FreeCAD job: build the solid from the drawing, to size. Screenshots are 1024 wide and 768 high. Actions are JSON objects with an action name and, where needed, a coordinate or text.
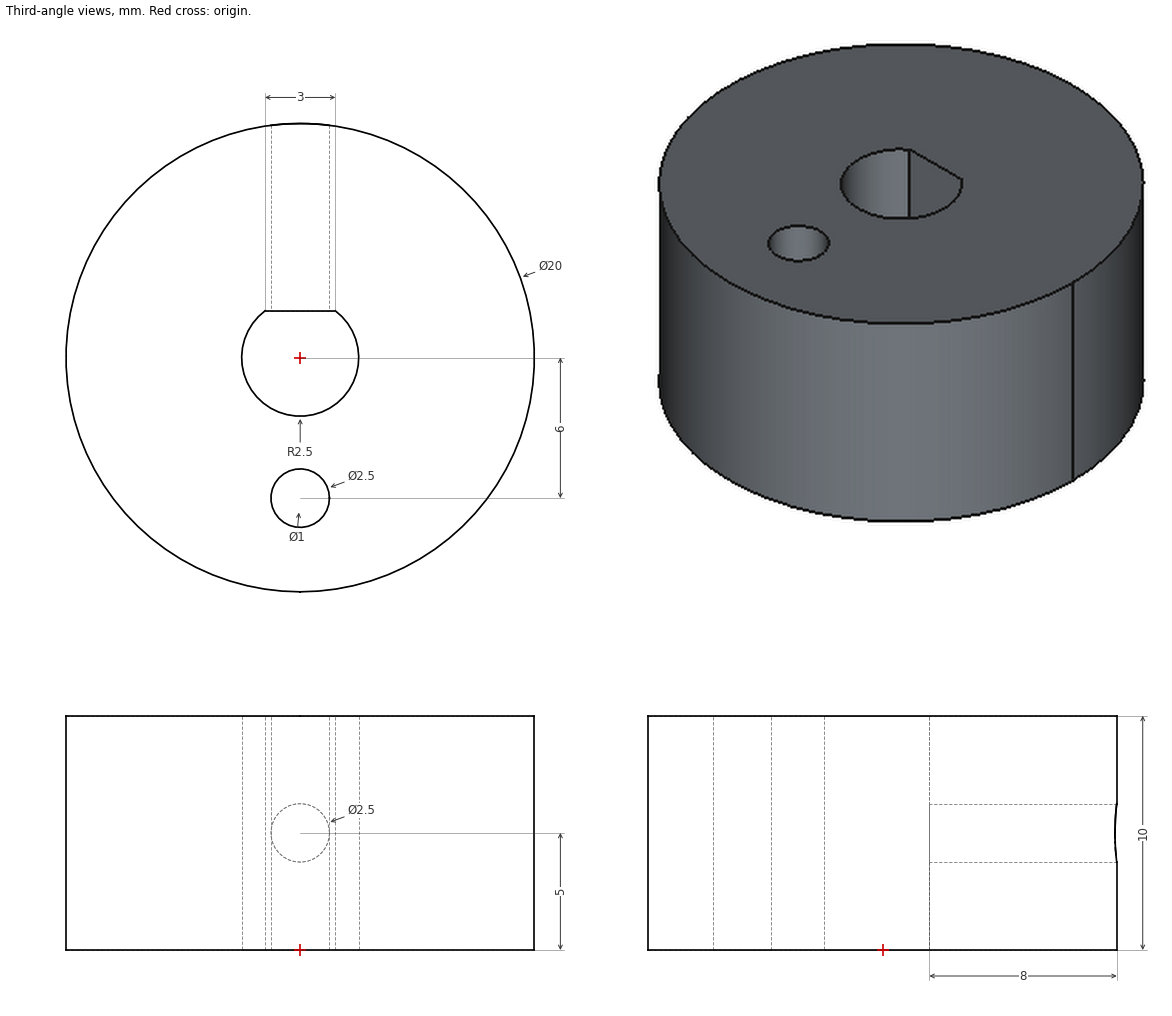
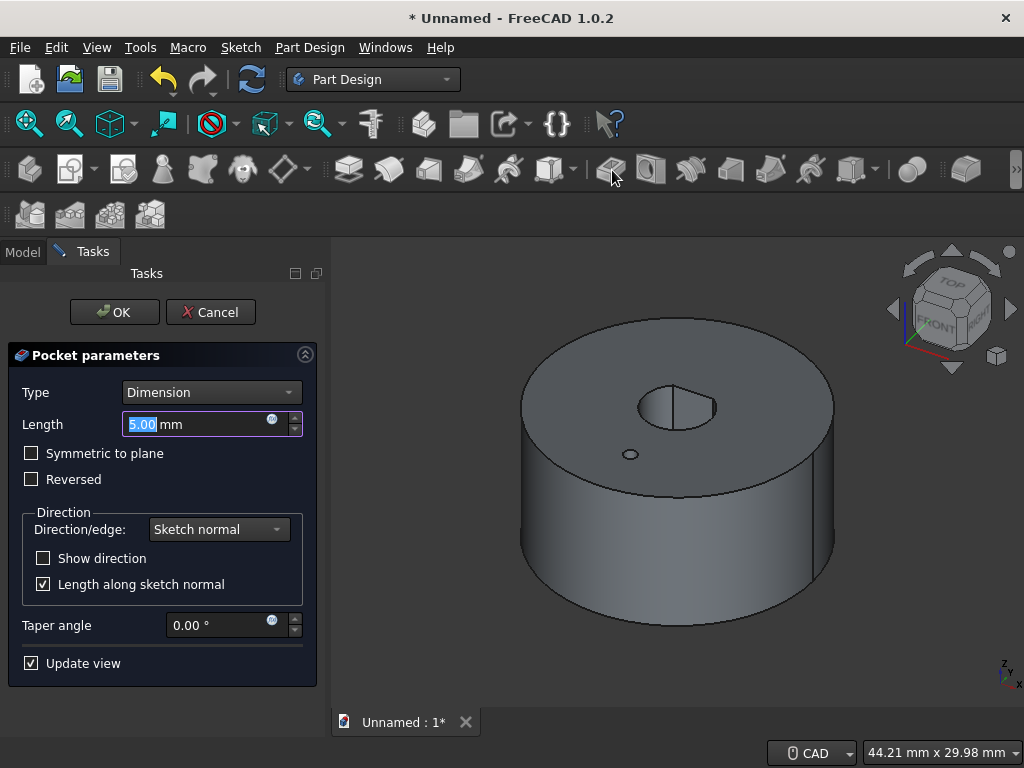
{"action": "left_click", "coordinate": [212, 392]}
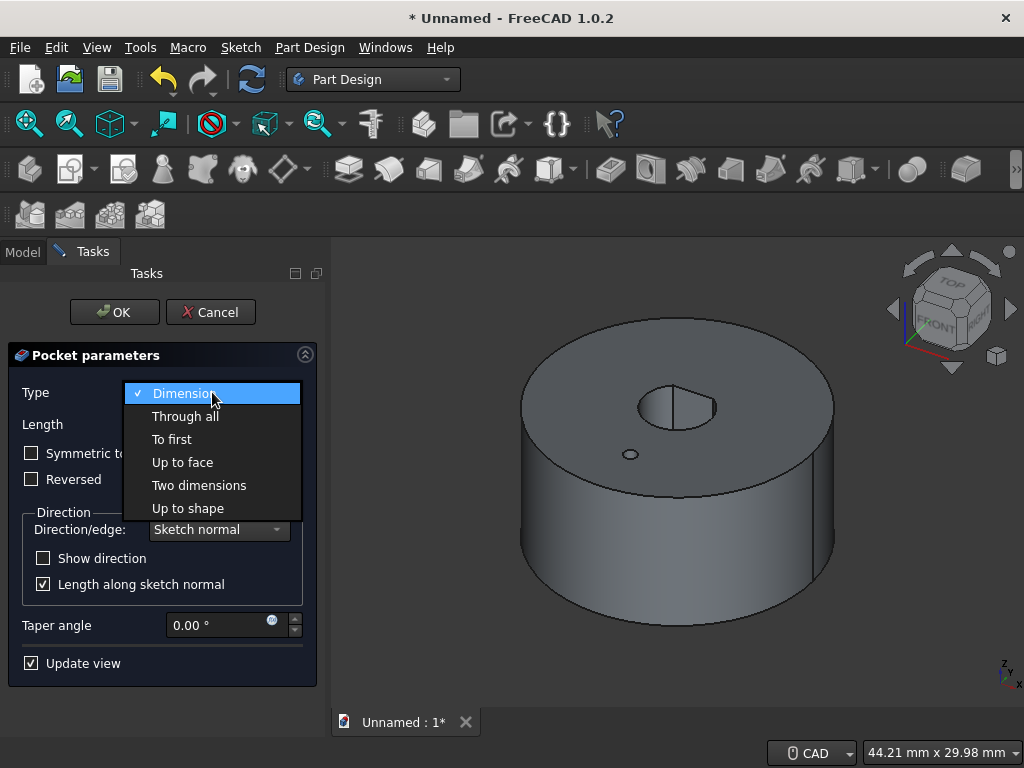
{"action": "left_click", "coordinate": [212, 416]}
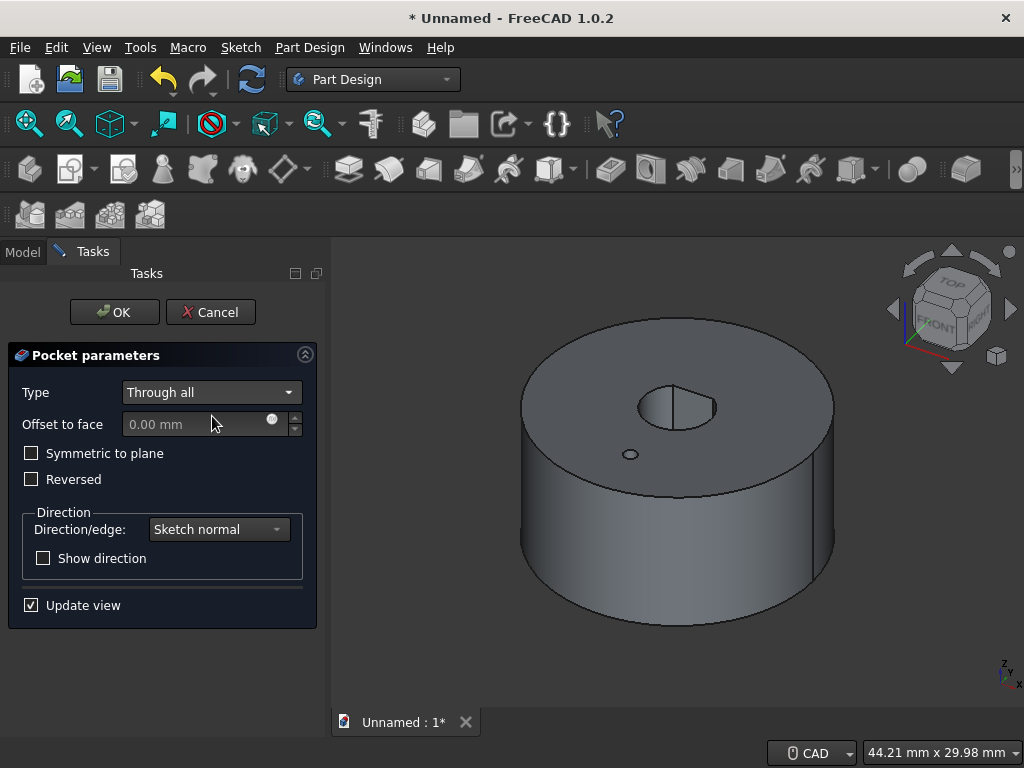
{"action": "left_click", "coordinate": [115, 312]}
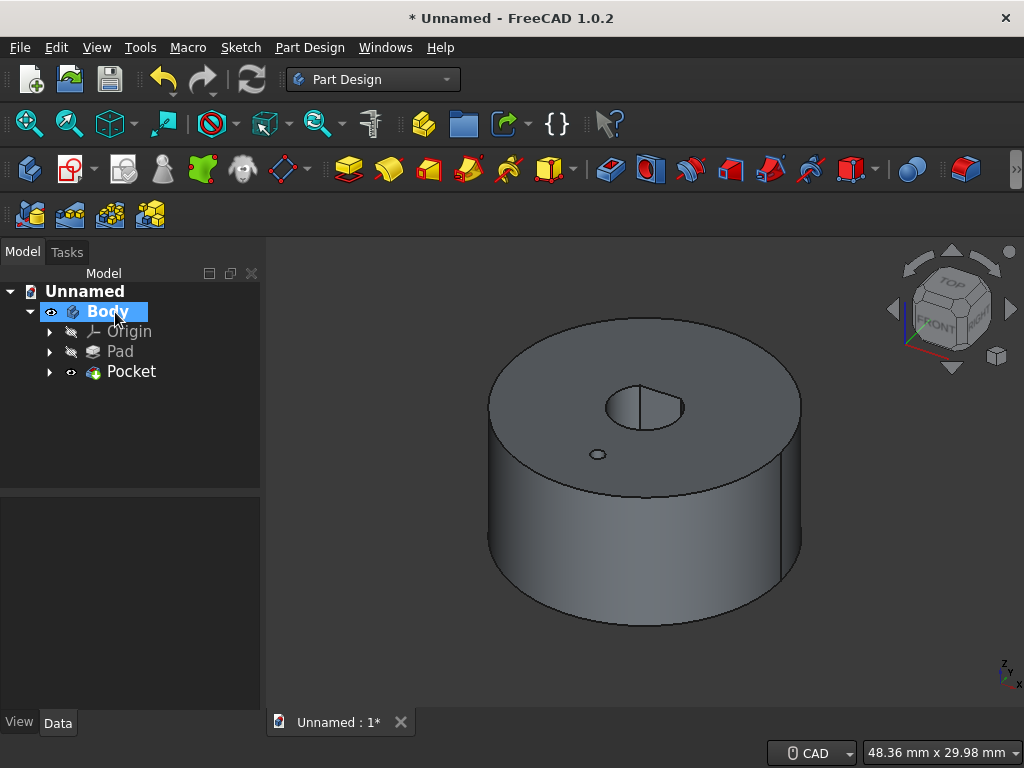
{"action": "left_click", "coordinate": [50, 332]}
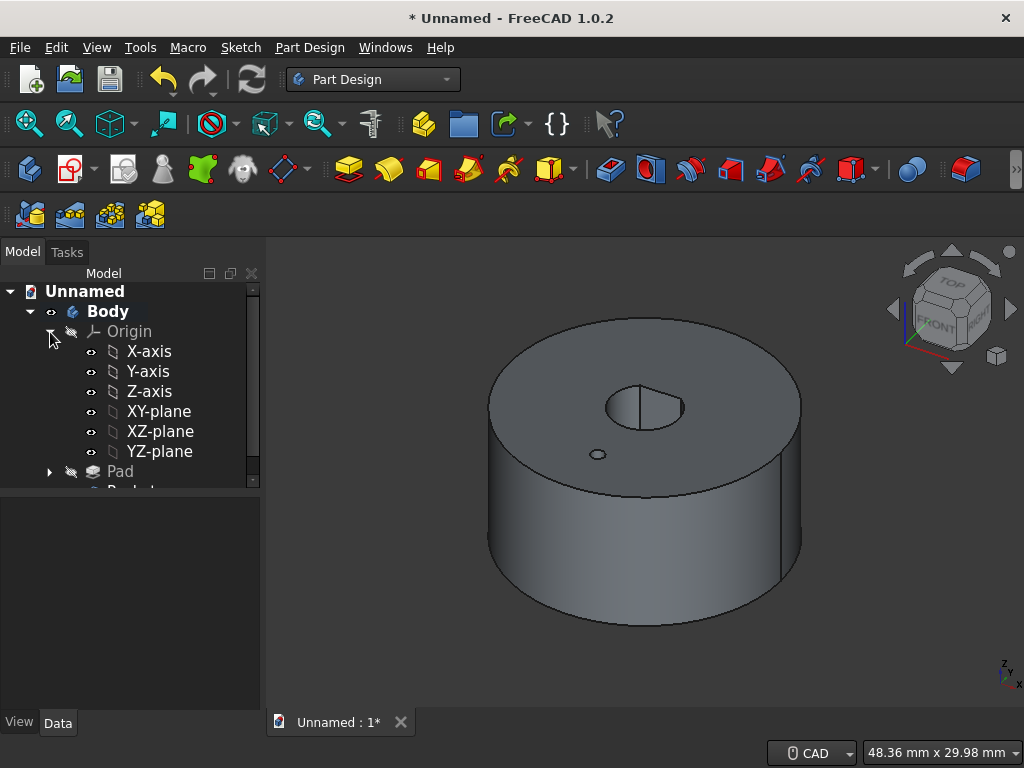
{"action": "left_click", "coordinate": [136, 432]}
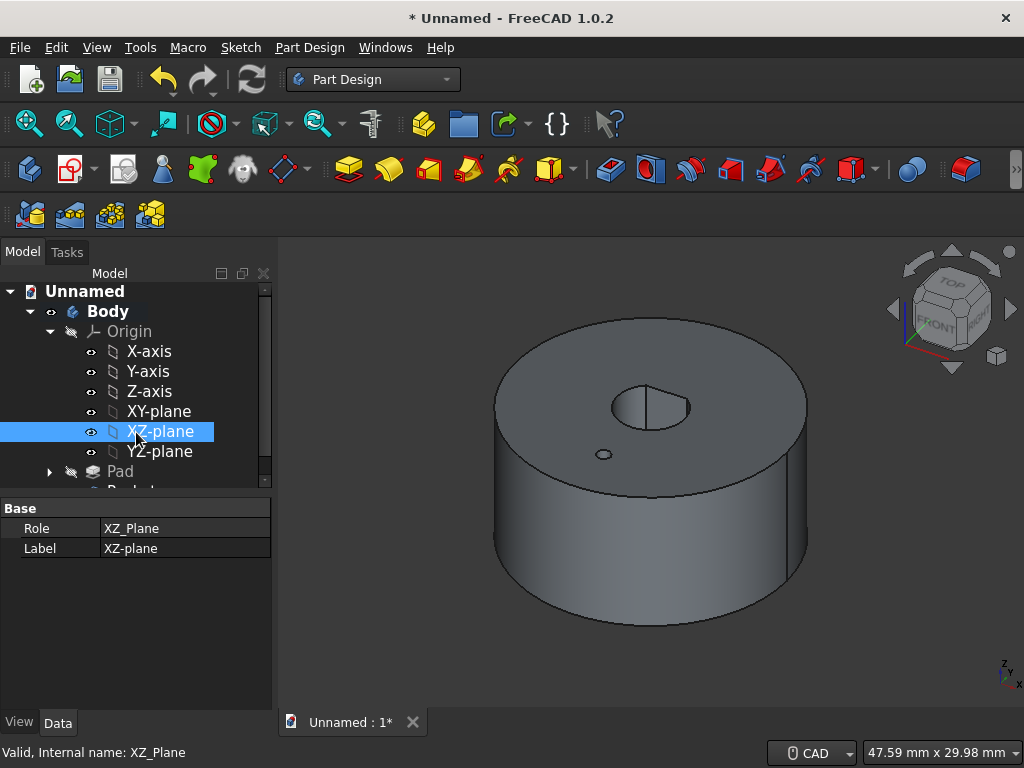
{"action": "left_click", "coordinate": [284, 170]}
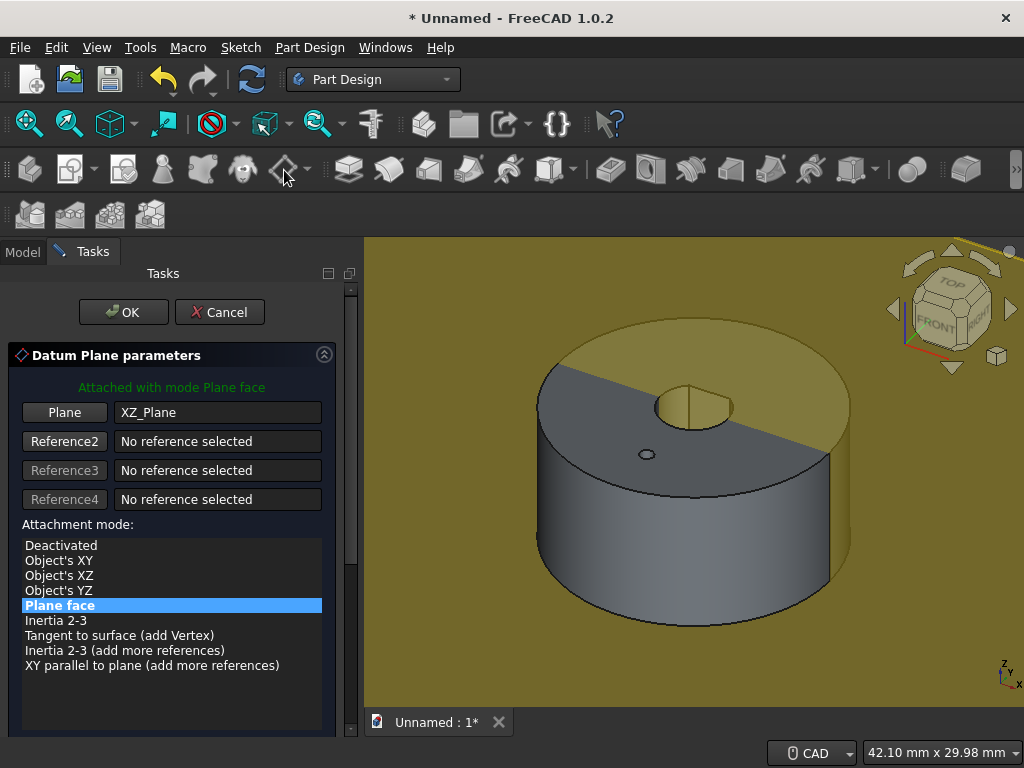
{"action": "scroll", "coordinate": [351, 510], "scroll_direction": "down", "scroll_amount": 3}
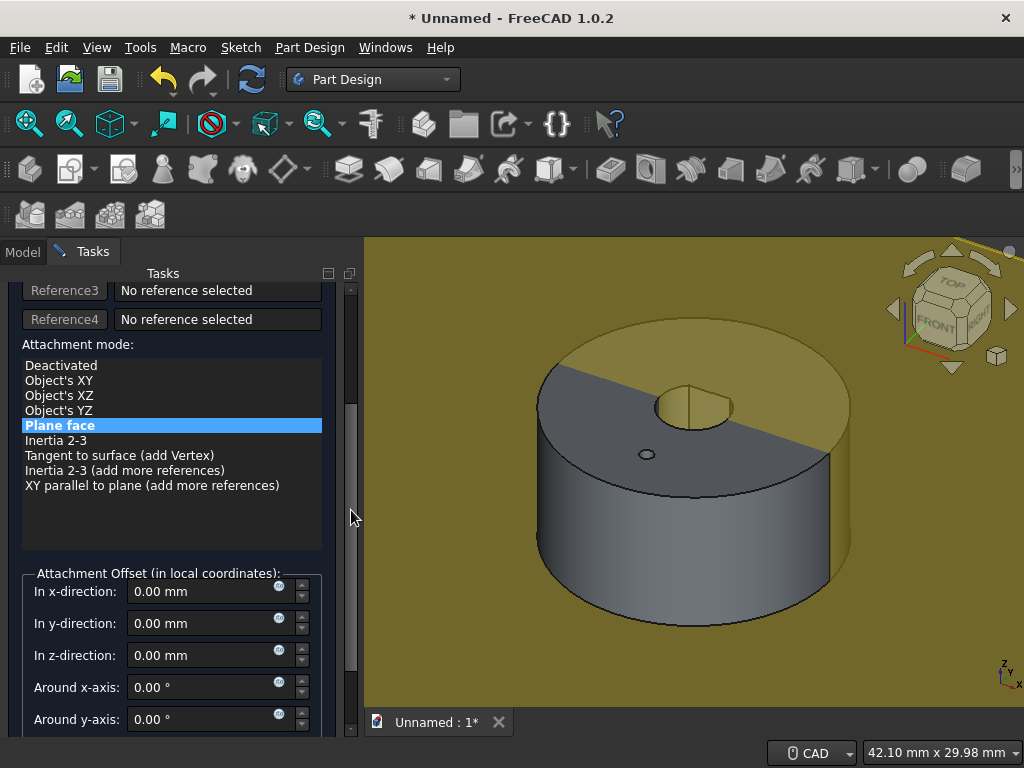
{"action": "triple_click", "coordinate": [210, 655]}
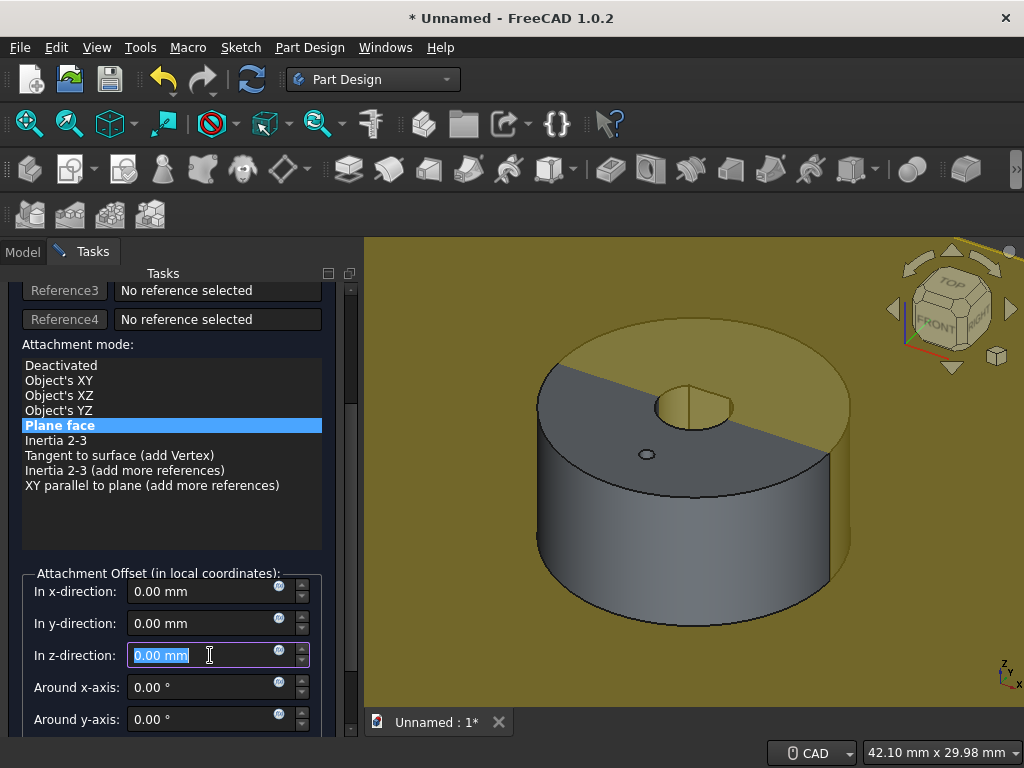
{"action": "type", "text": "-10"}
{"action": "key", "text": "Tab"}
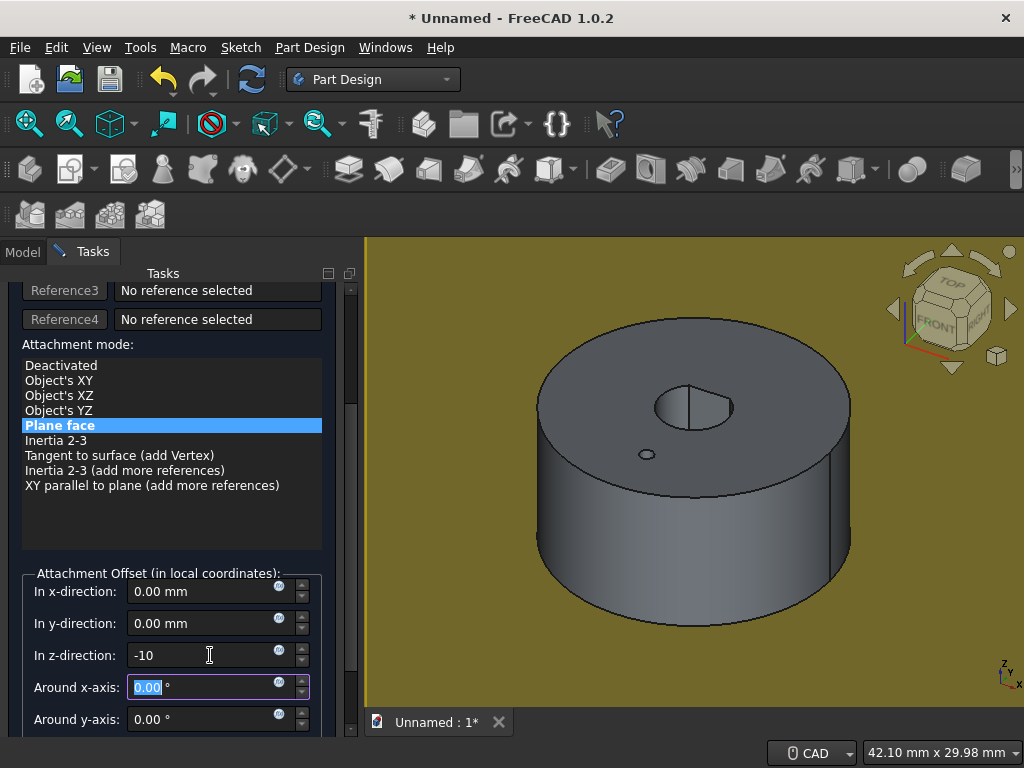
{"action": "scroll", "coordinate": [351, 510], "scroll_direction": "up", "scroll_amount": 4}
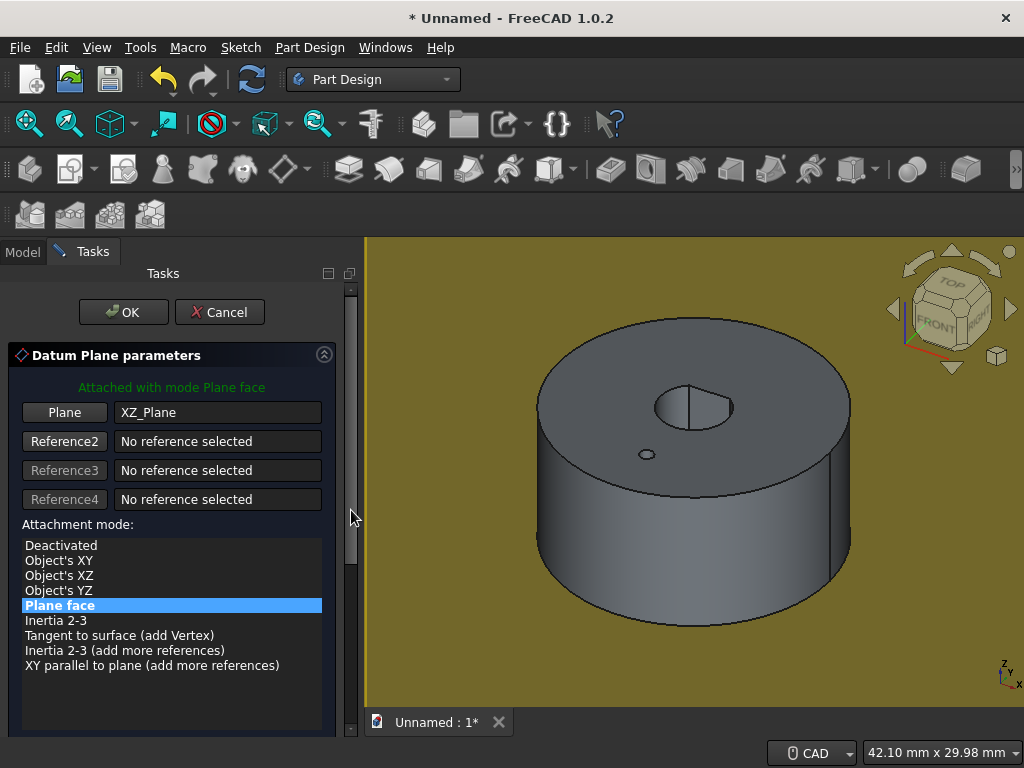
{"action": "left_click", "coordinate": [124, 312]}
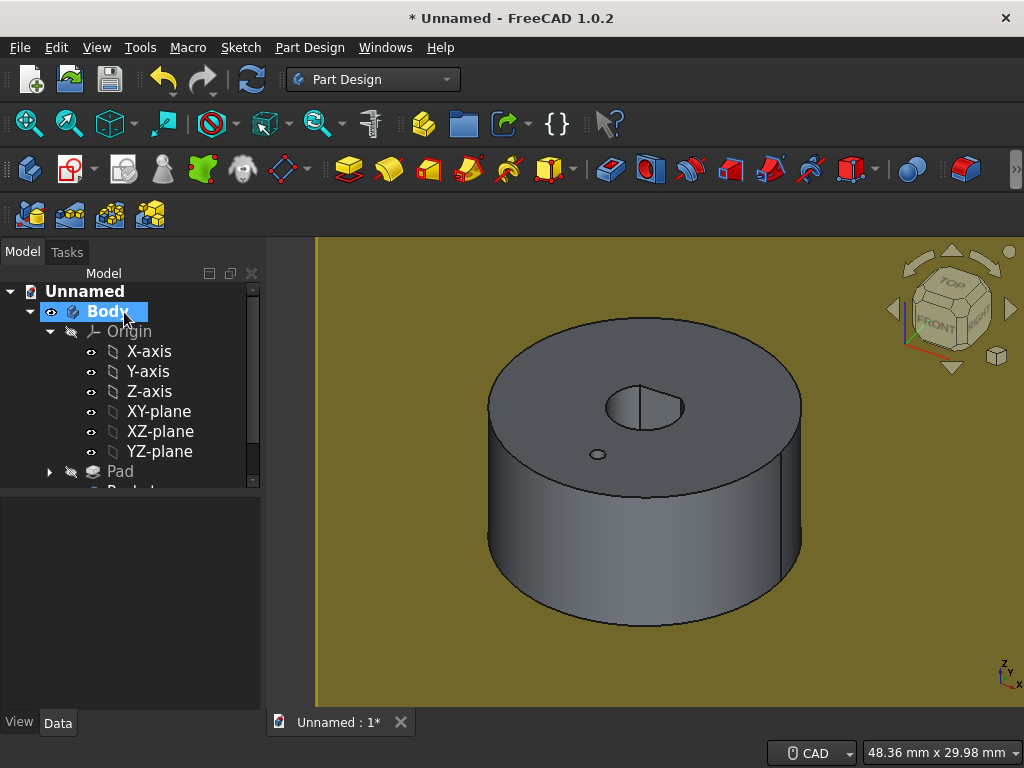
{"action": "scroll", "coordinate": [100, 387], "scroll_direction": "down", "scroll_amount": 3}